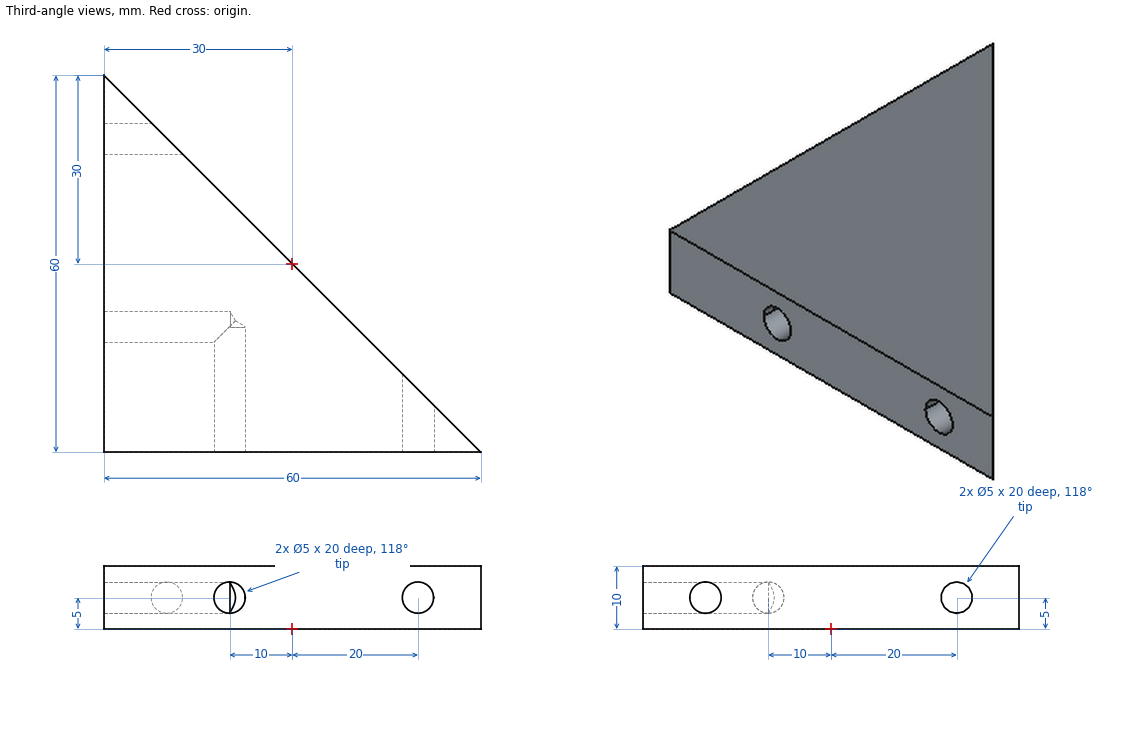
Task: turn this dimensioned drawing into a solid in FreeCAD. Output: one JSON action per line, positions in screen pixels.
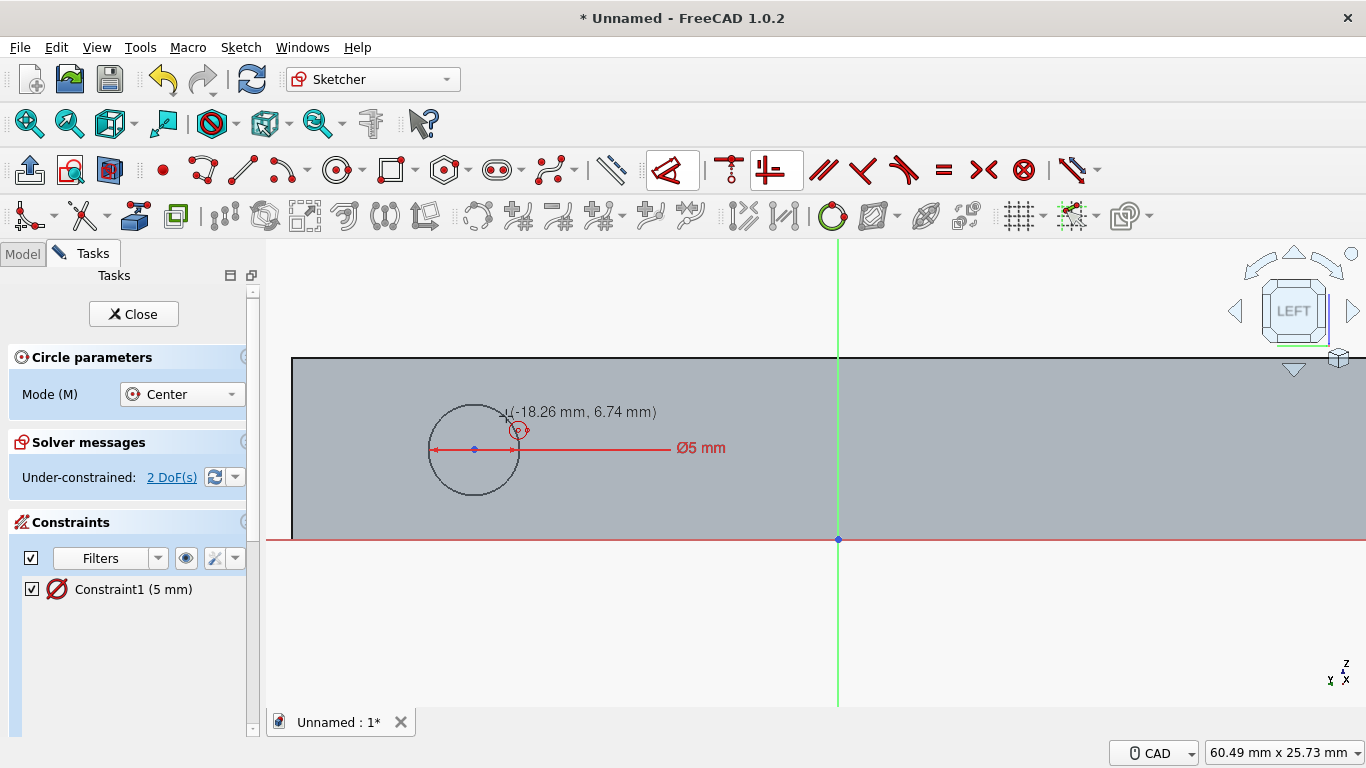
{"action": "left_click", "coordinate": [1020, 449]}
{"action": "mouse_move", "coordinate": [1052, 416]}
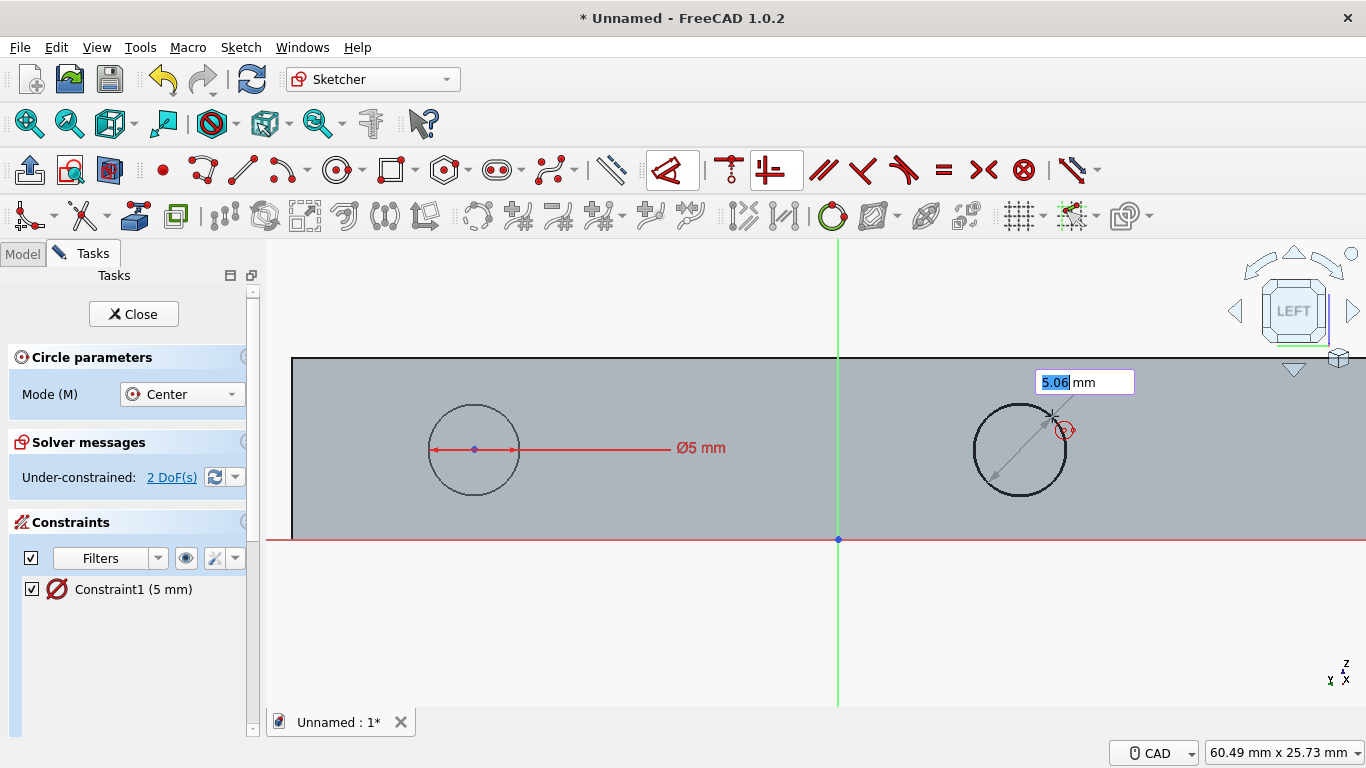
{"action": "type", "text": "5"}
{"action": "key", "text": "Return"}
{"action": "key", "text": "Escape"}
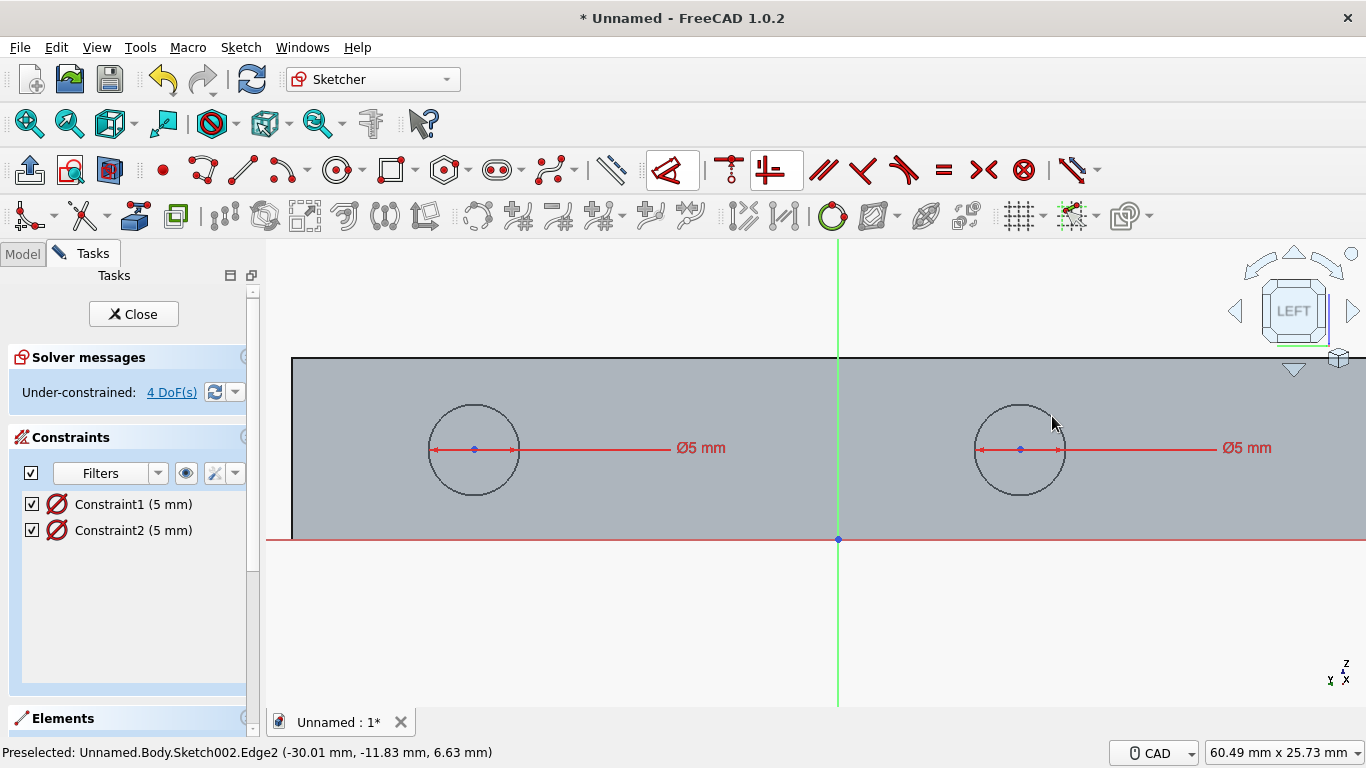
{"action": "left_click", "coordinate": [474, 450]}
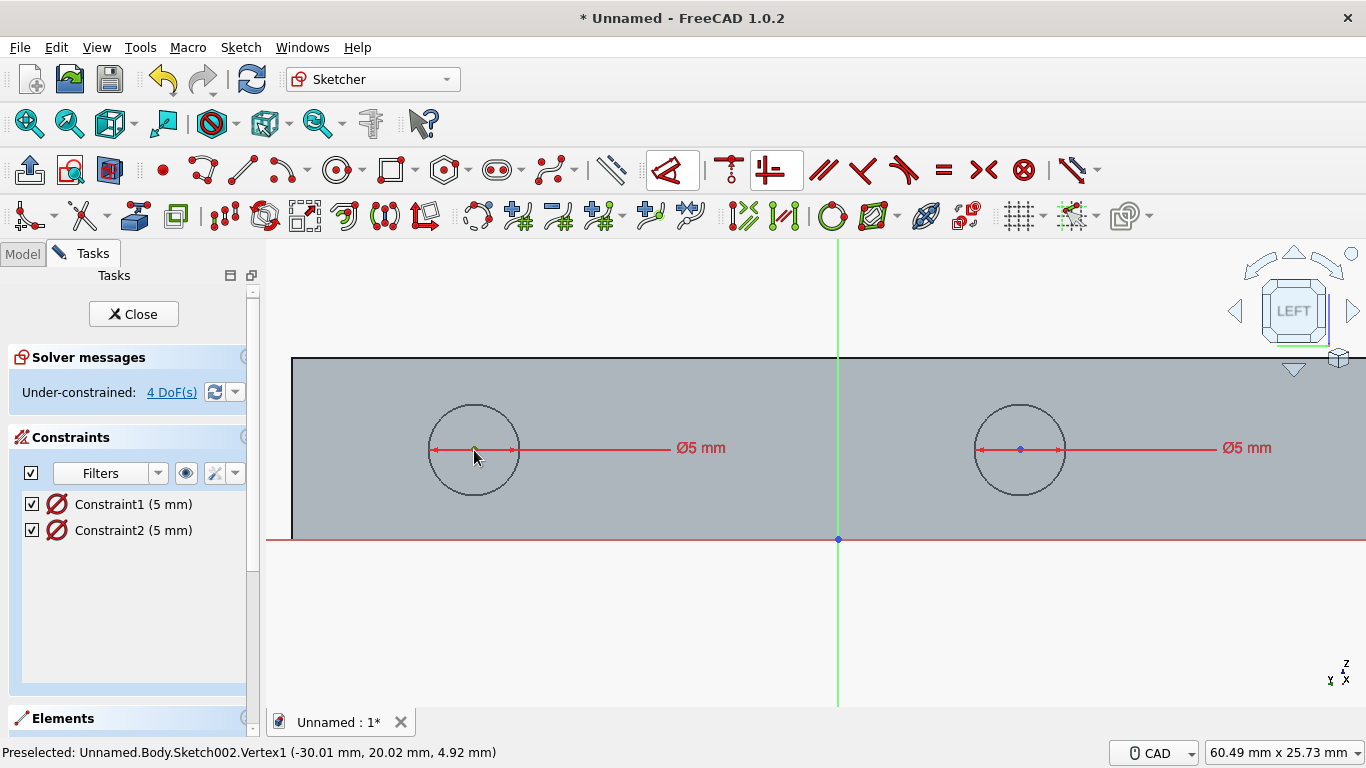
{"action": "key", "text": "i"}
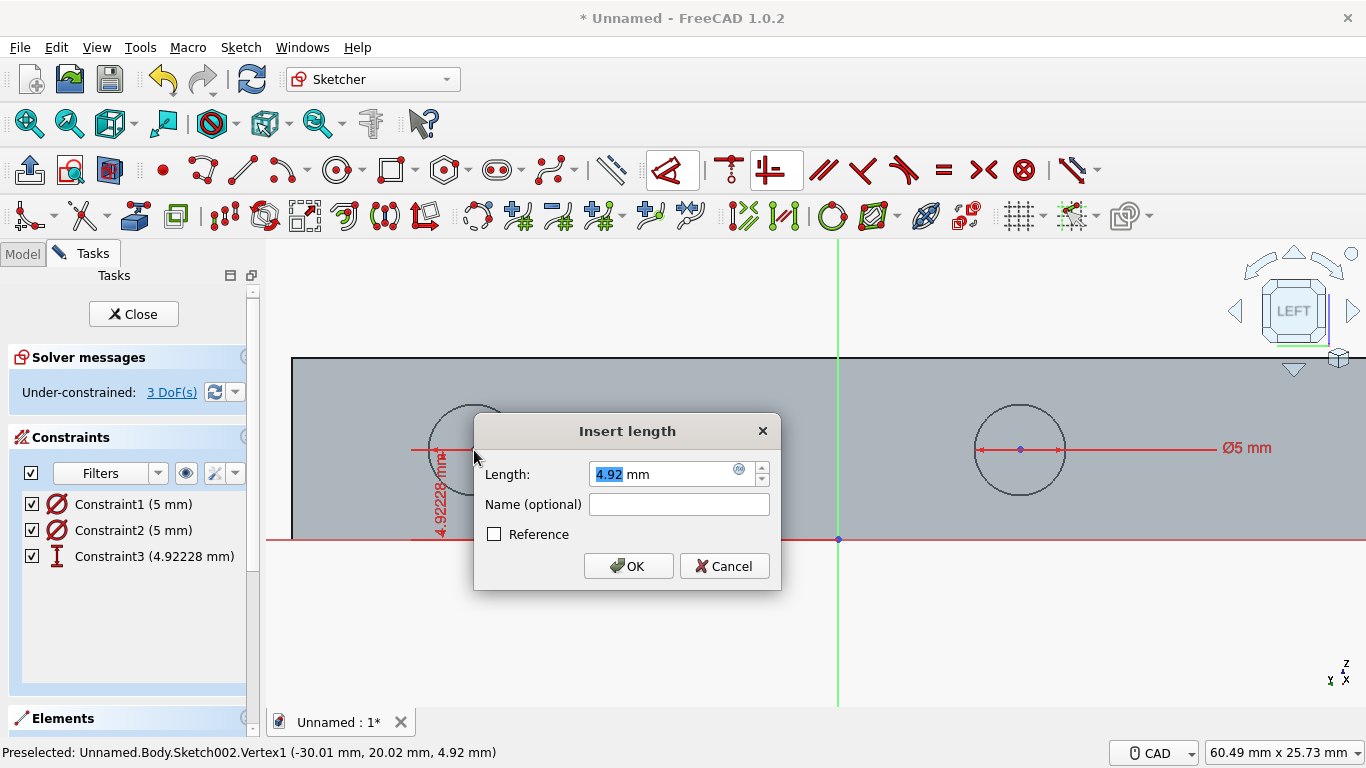
{"action": "type", "text": "5"}
{"action": "key", "text": "Return"}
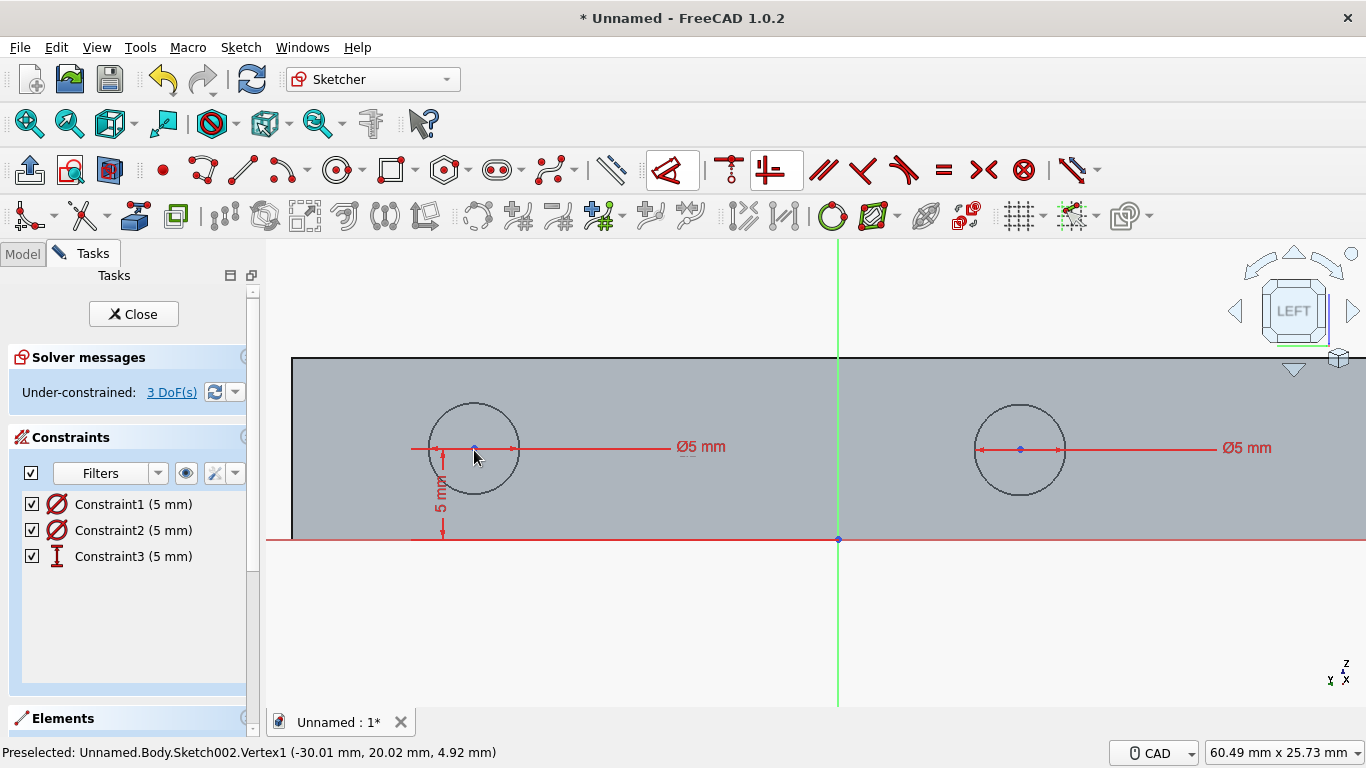
{"action": "left_click", "coordinate": [1020, 450]}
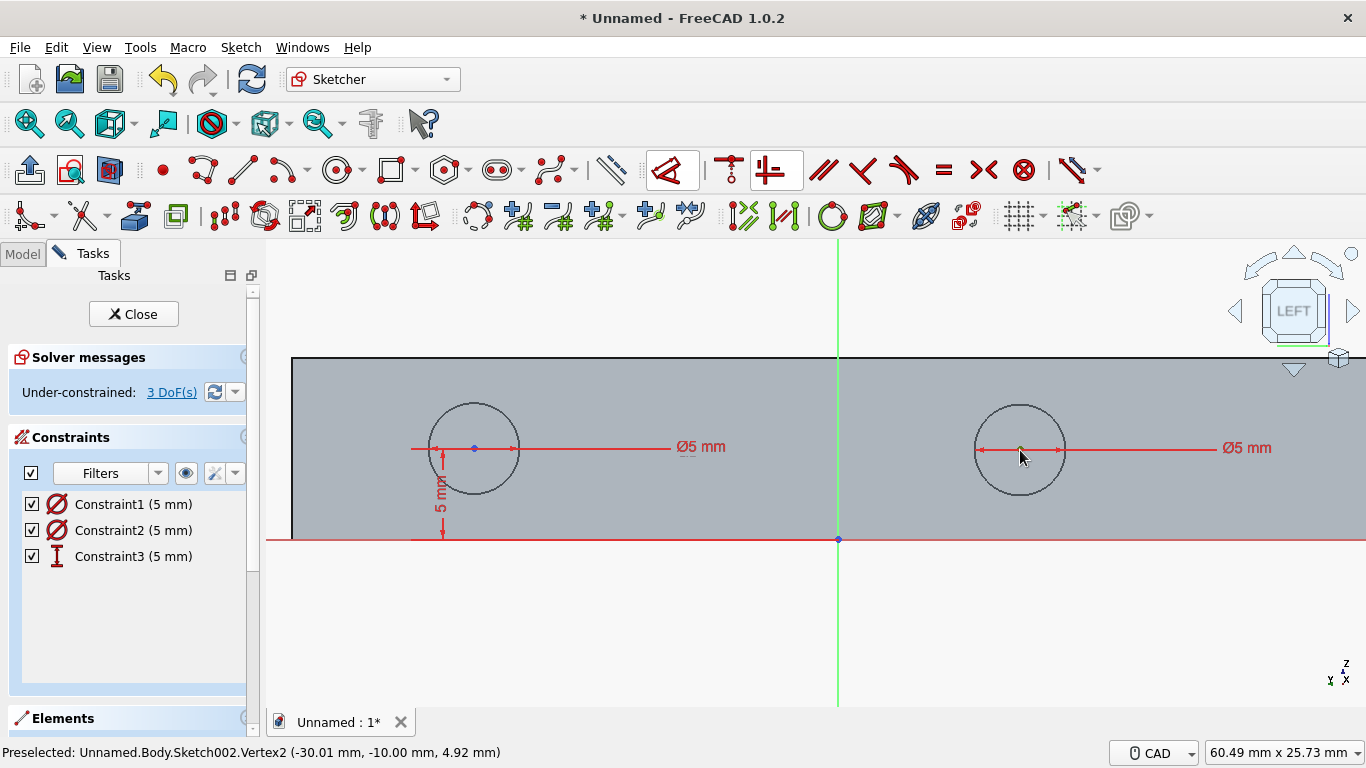
{"action": "key", "text": "i"}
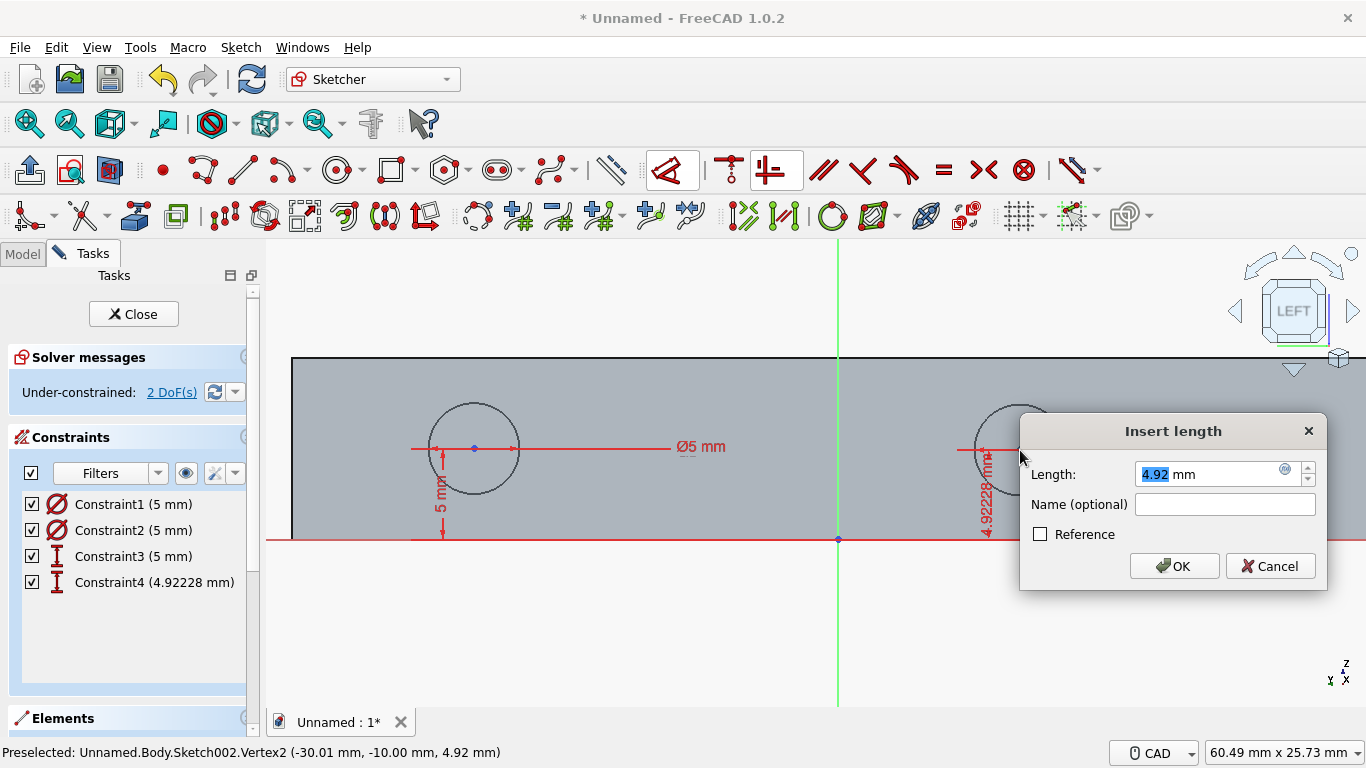
{"action": "type", "text": "5"}
{"action": "key", "text": "Return"}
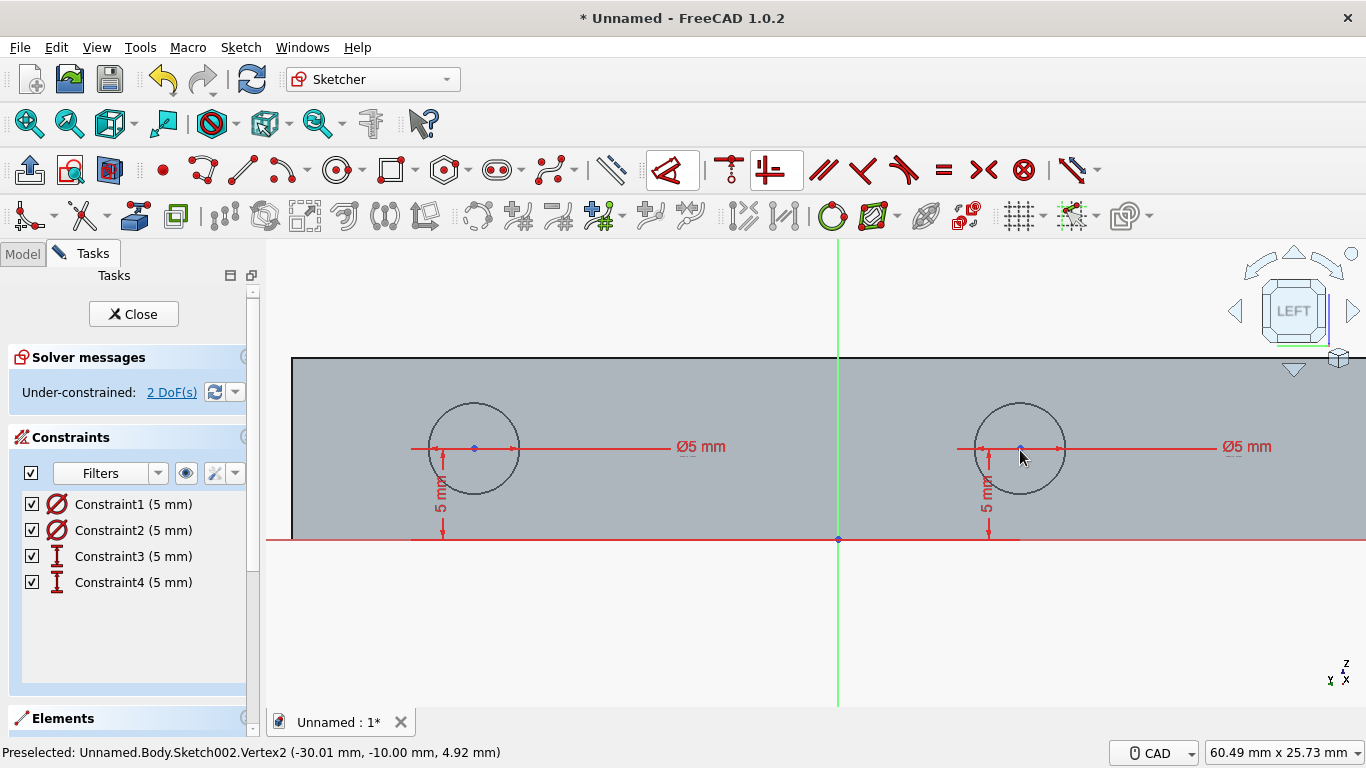
{"action": "left_click", "coordinate": [474, 449]}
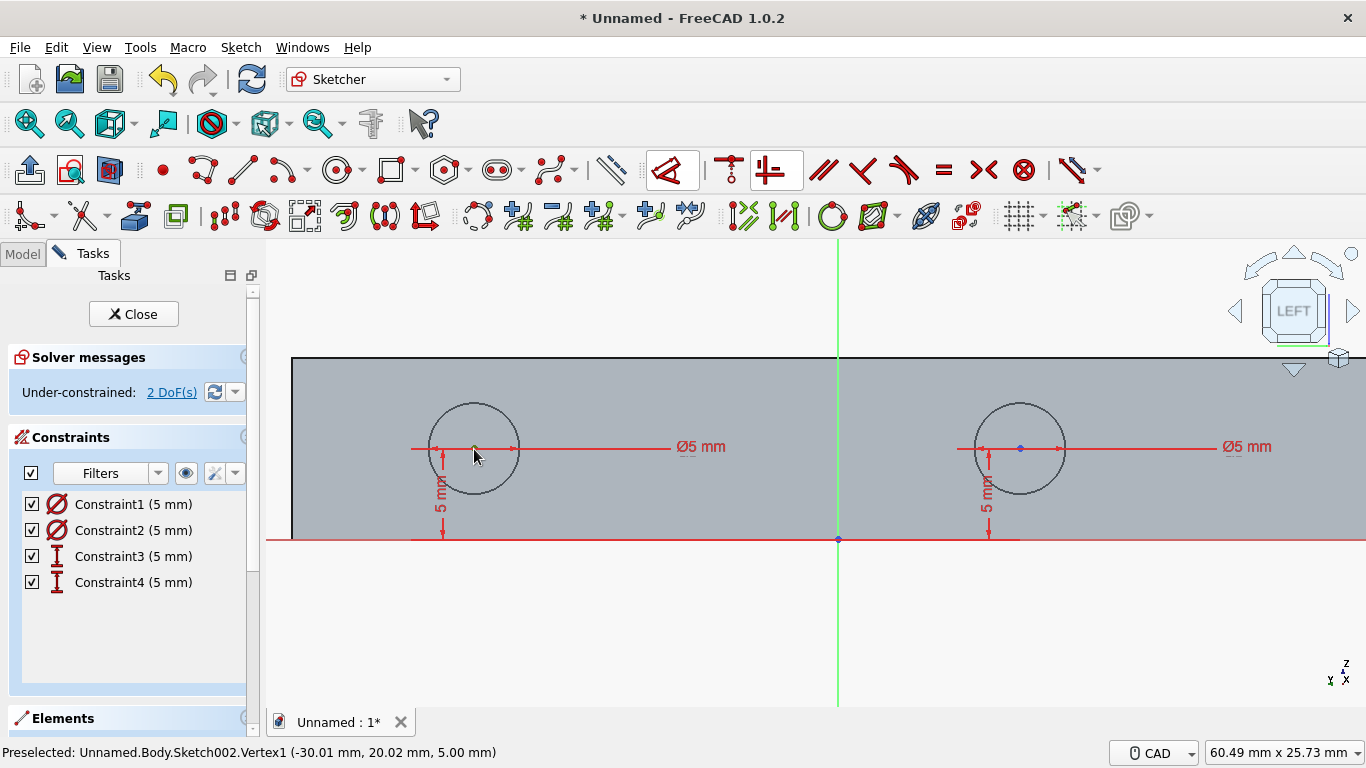
{"action": "key", "text": "l"}